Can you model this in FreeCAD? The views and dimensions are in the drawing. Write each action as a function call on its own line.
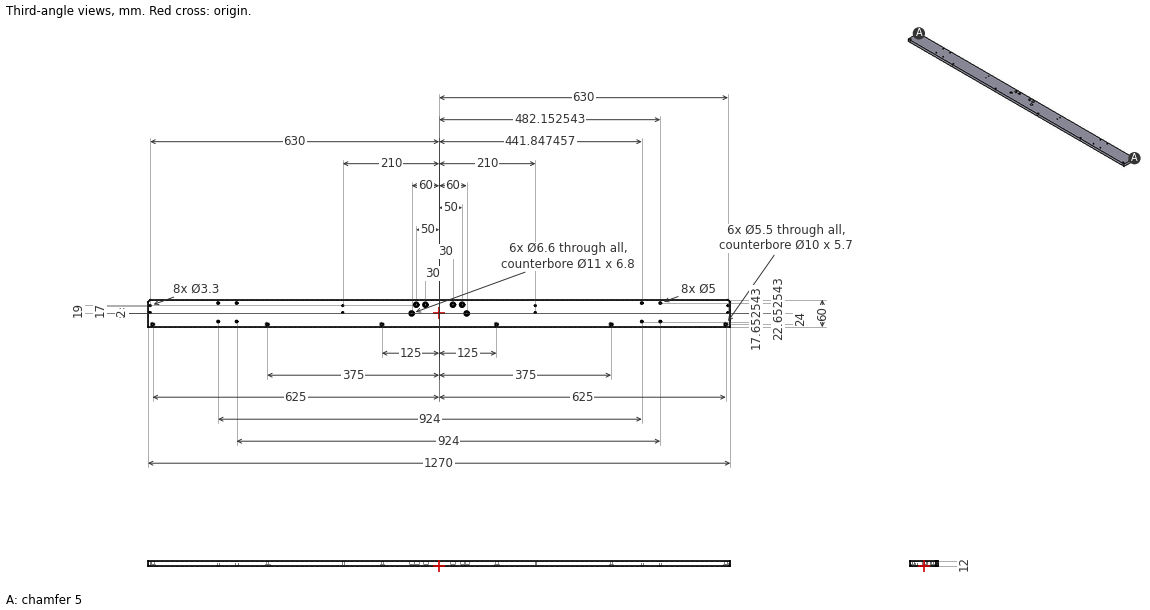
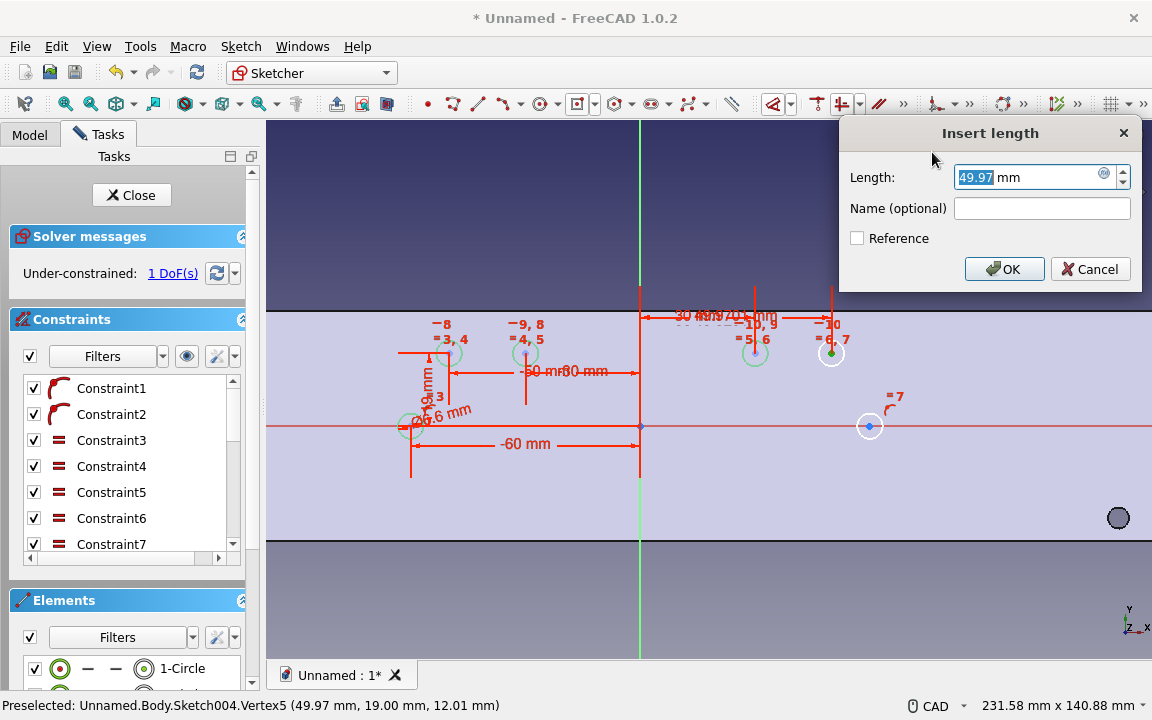
text(50)
key(Return)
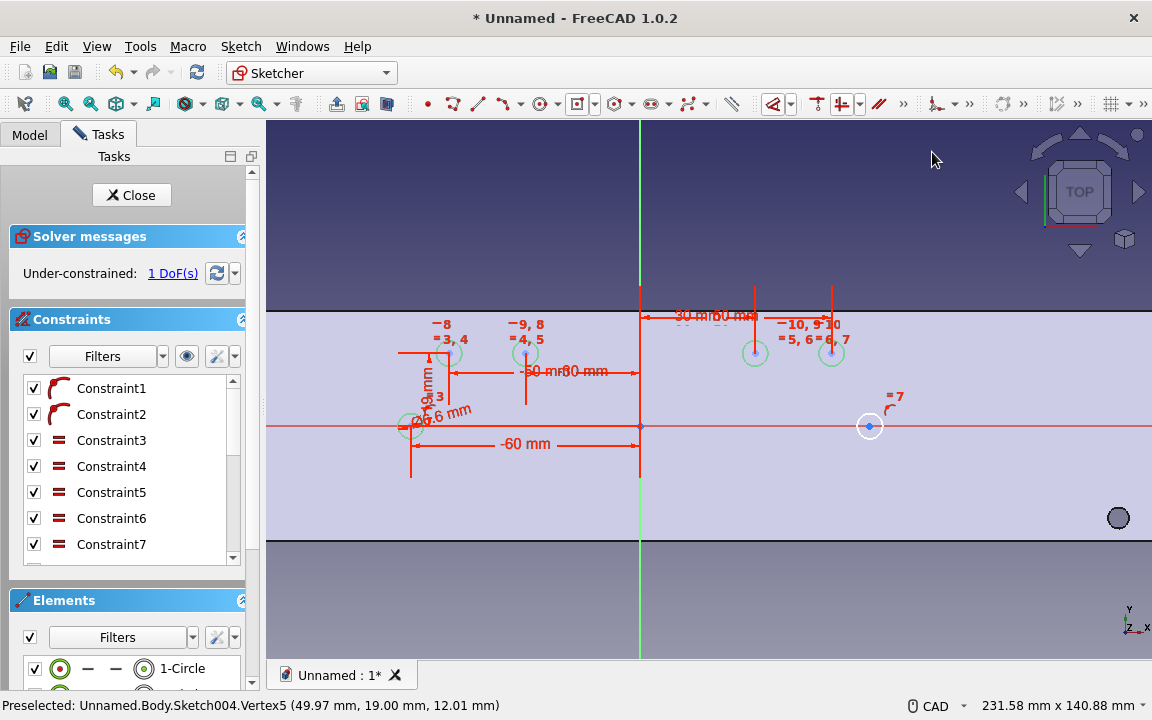
click(870, 426)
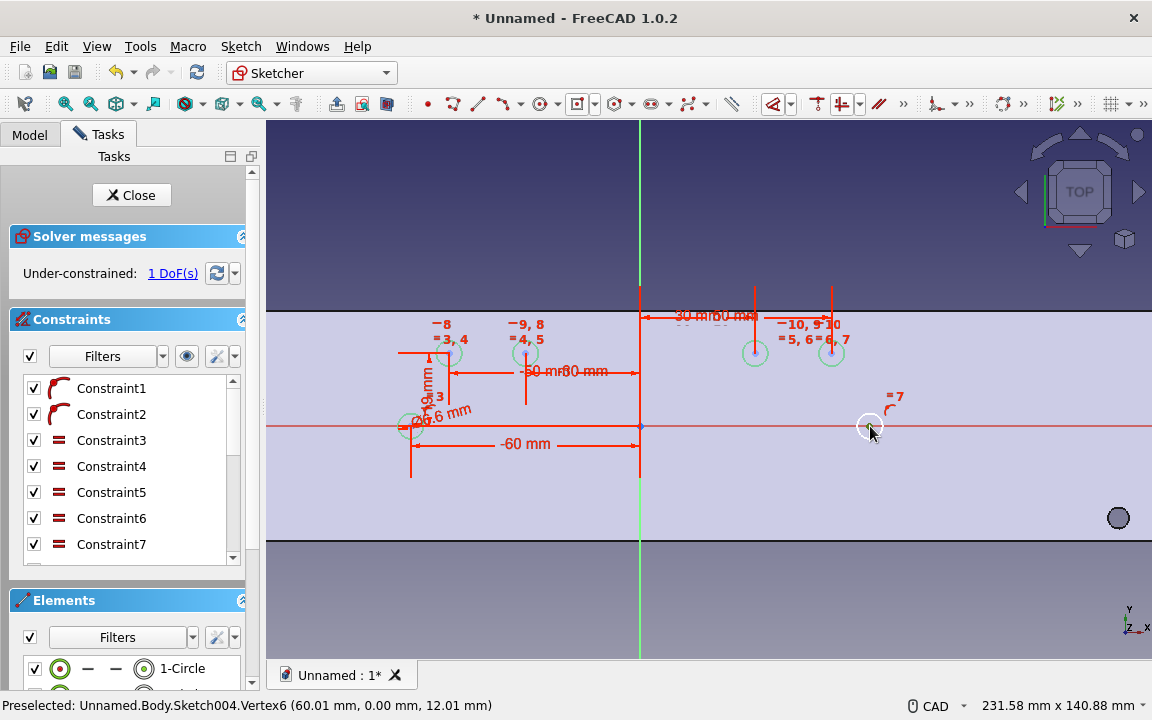
key(l)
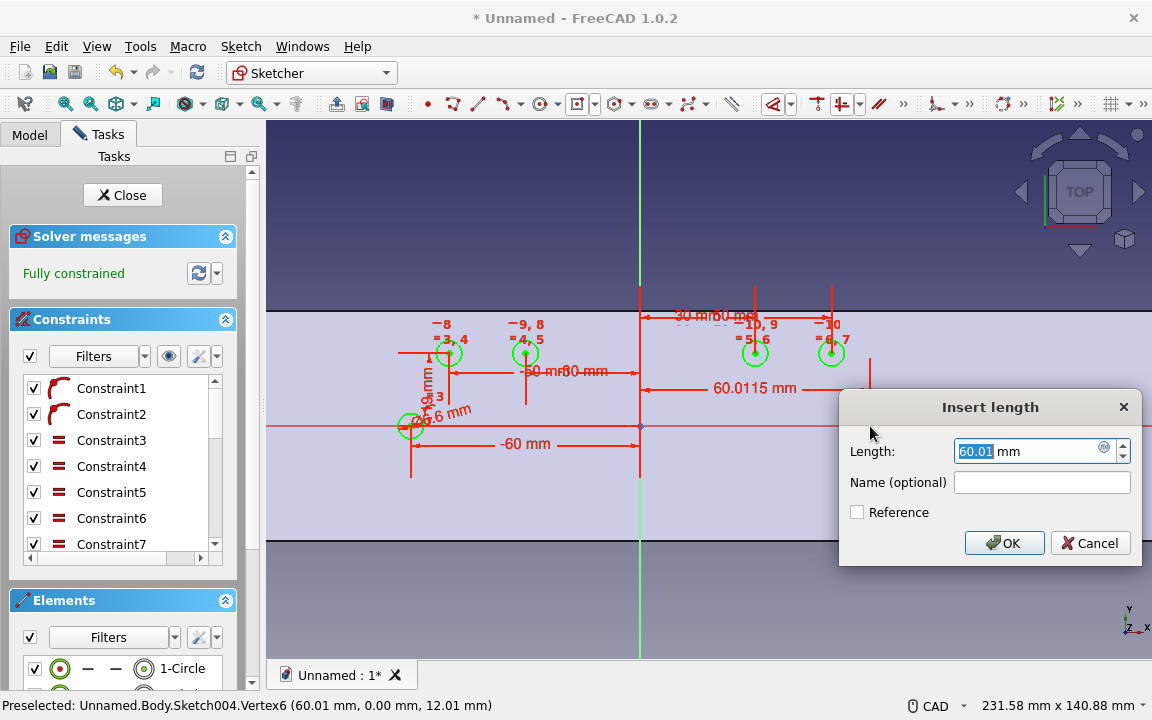
text(60)
key(Return)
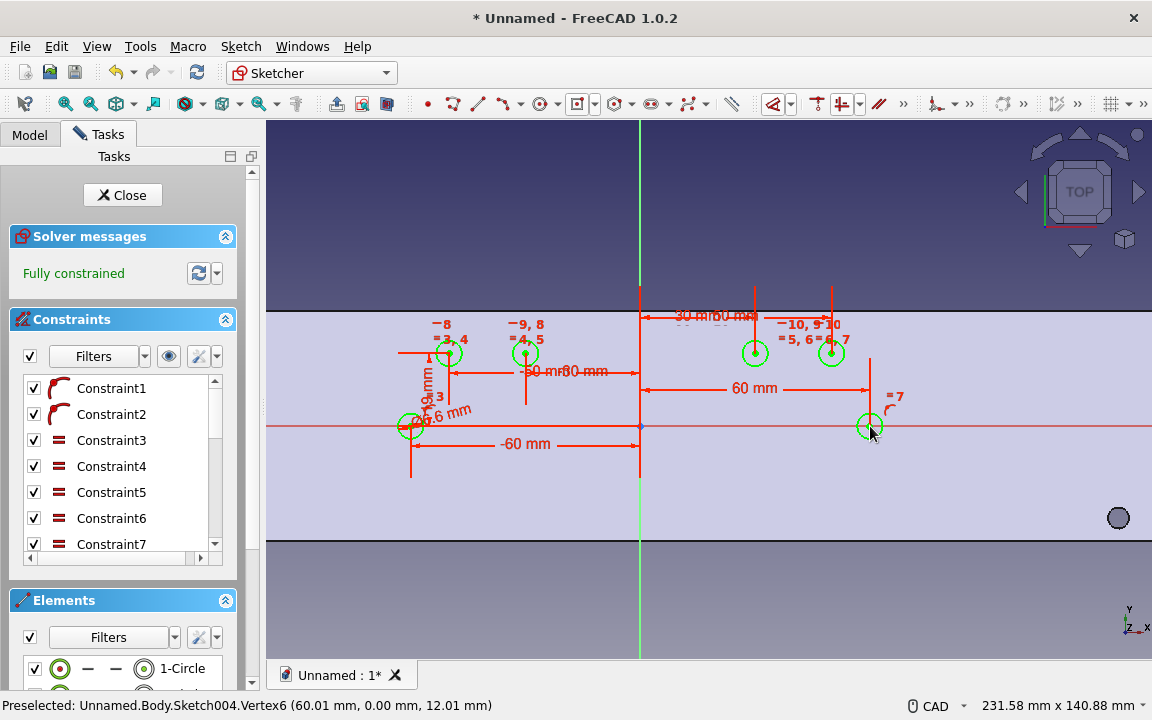
click(123, 195)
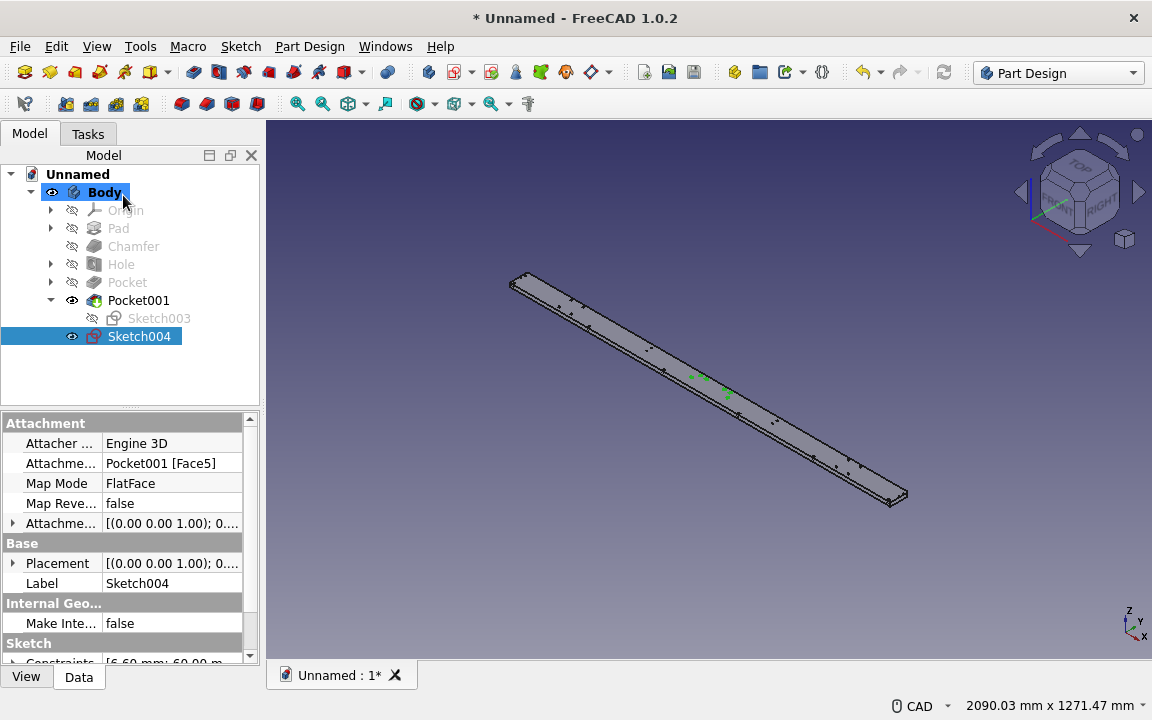
click(219, 72)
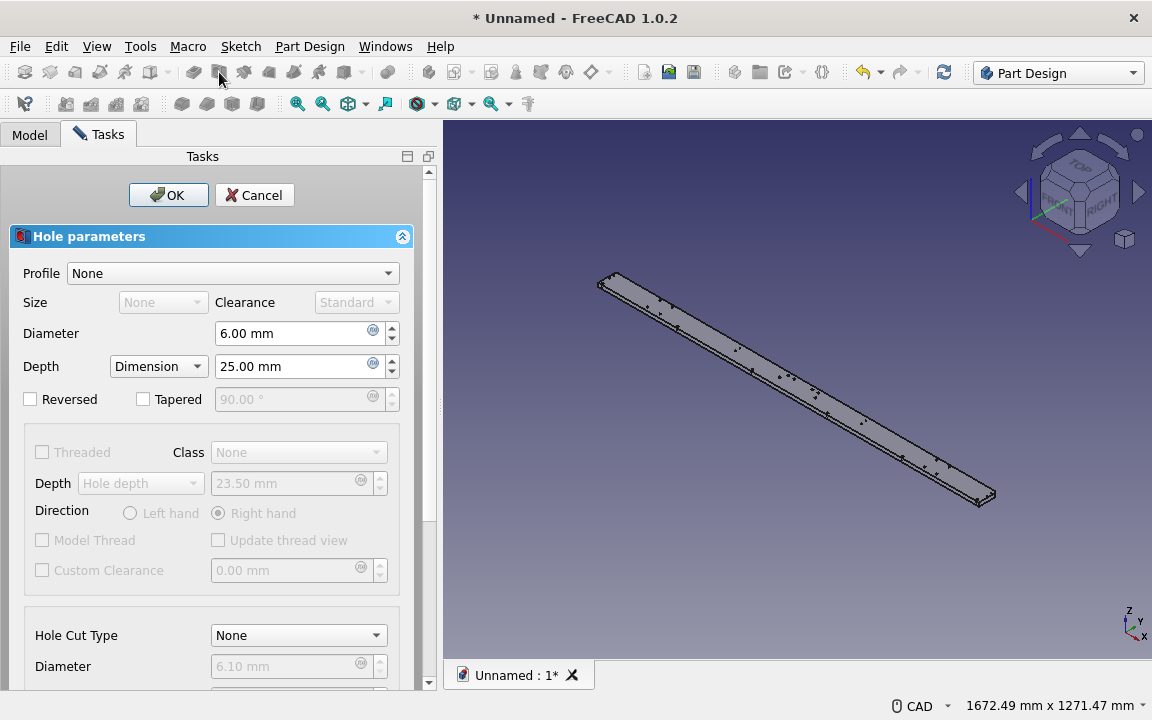
triple_click(300, 334)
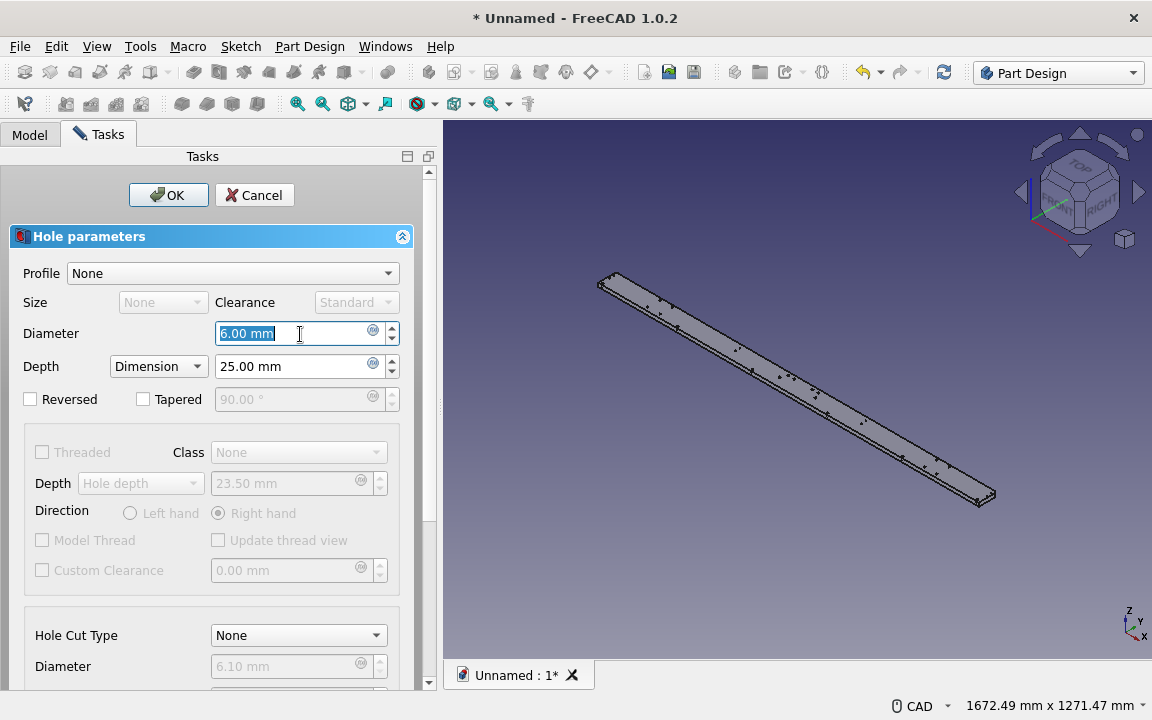
text(6.6)
key(Tab)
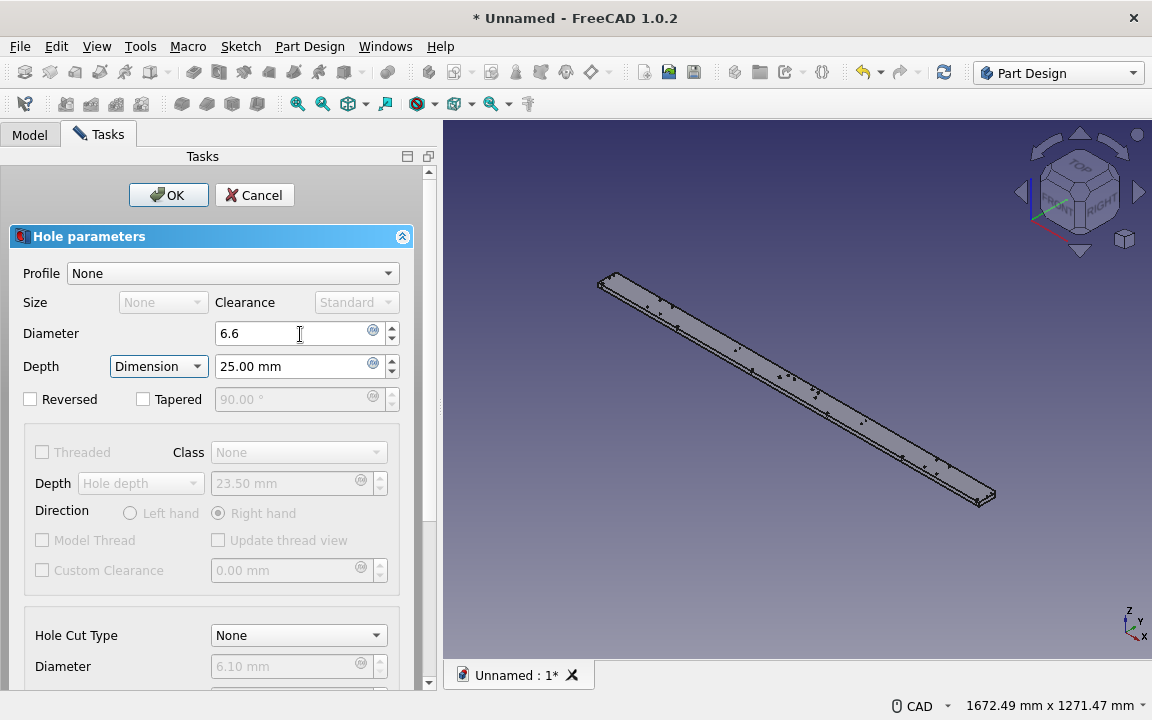
click(160, 366)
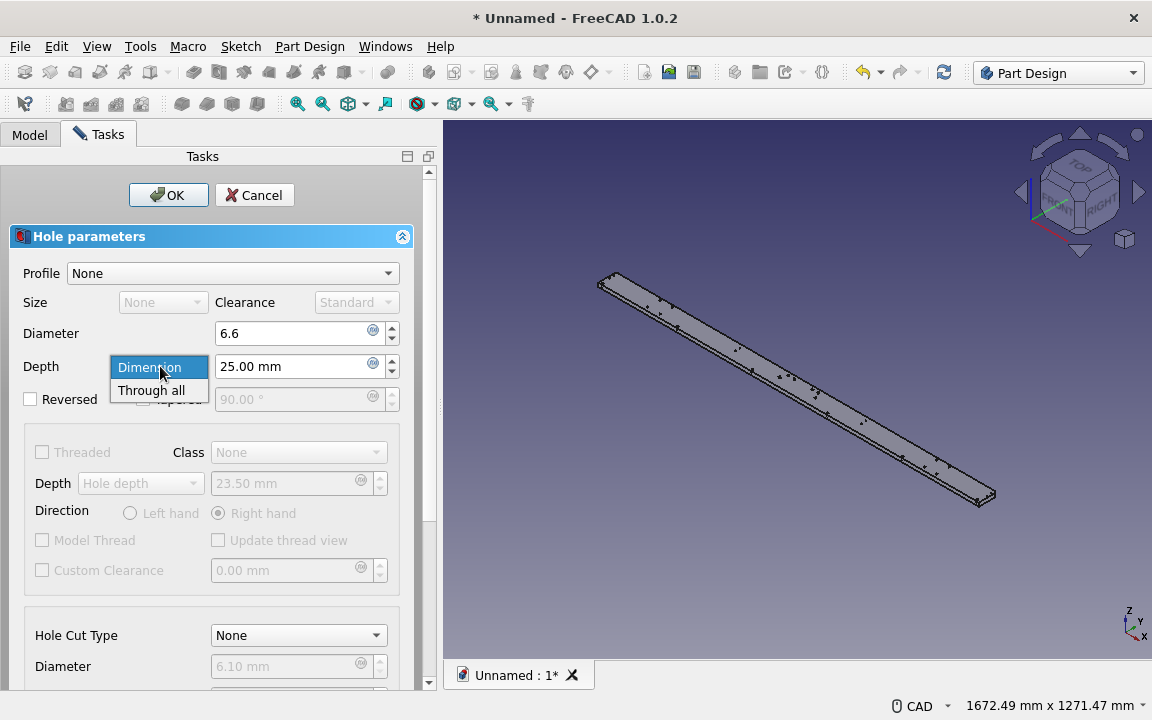
click(158, 390)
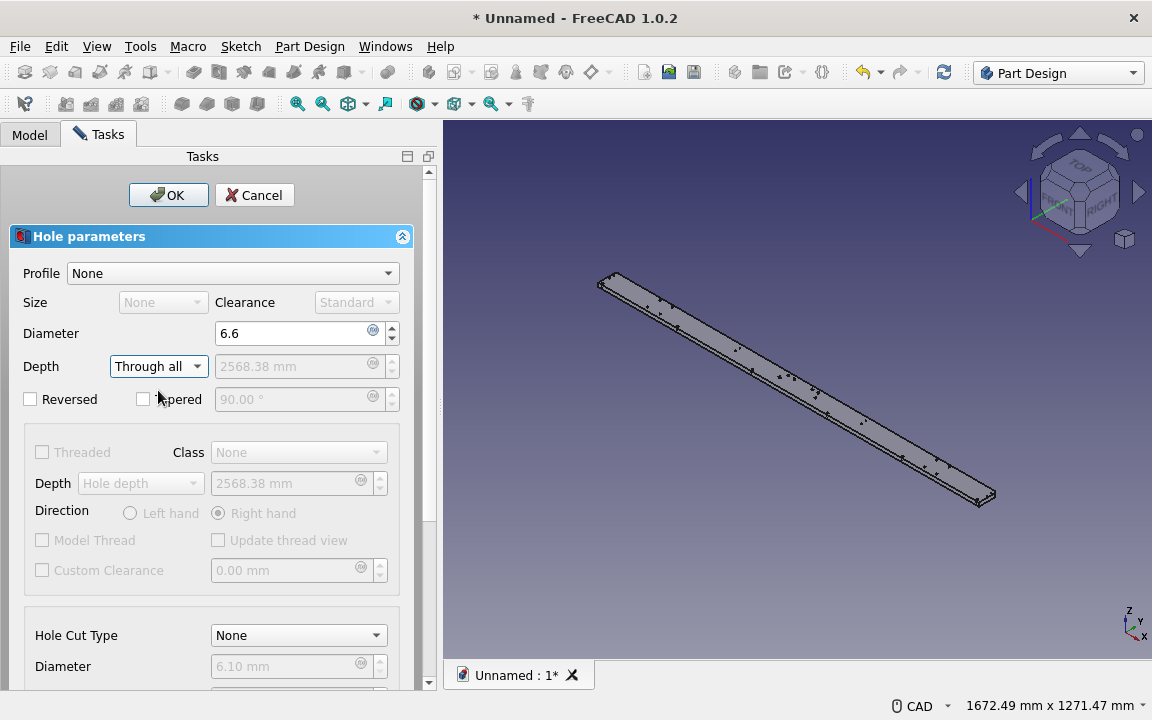
click(300, 636)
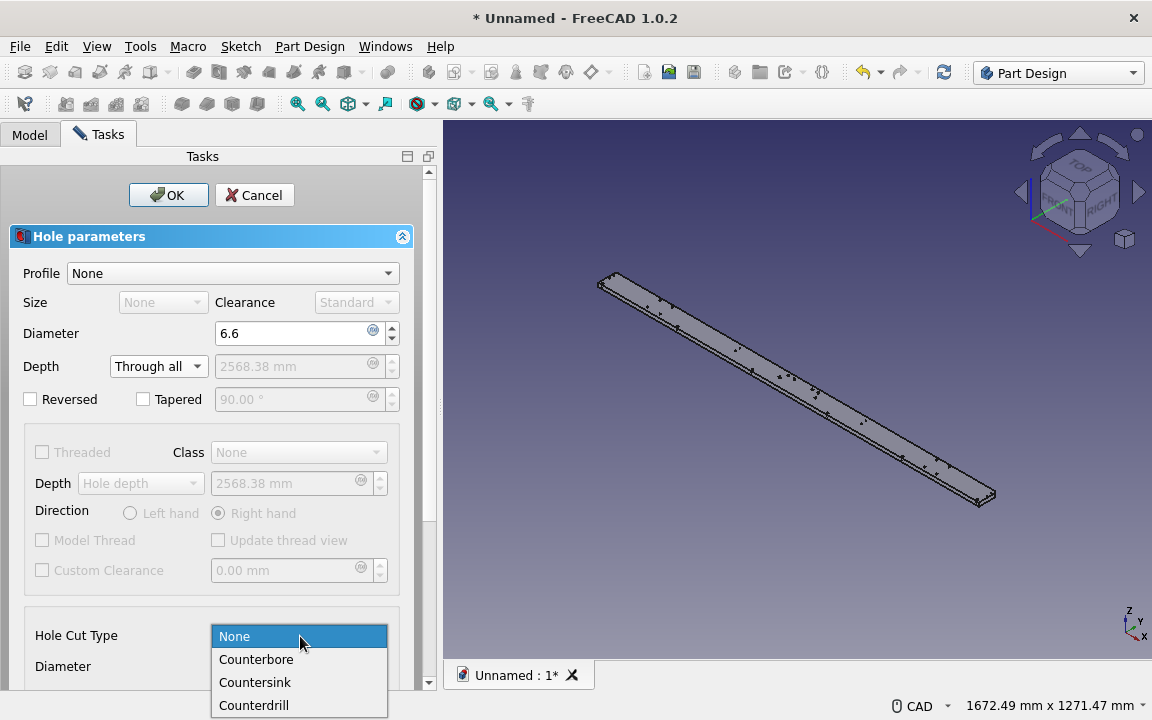
click(298, 660)